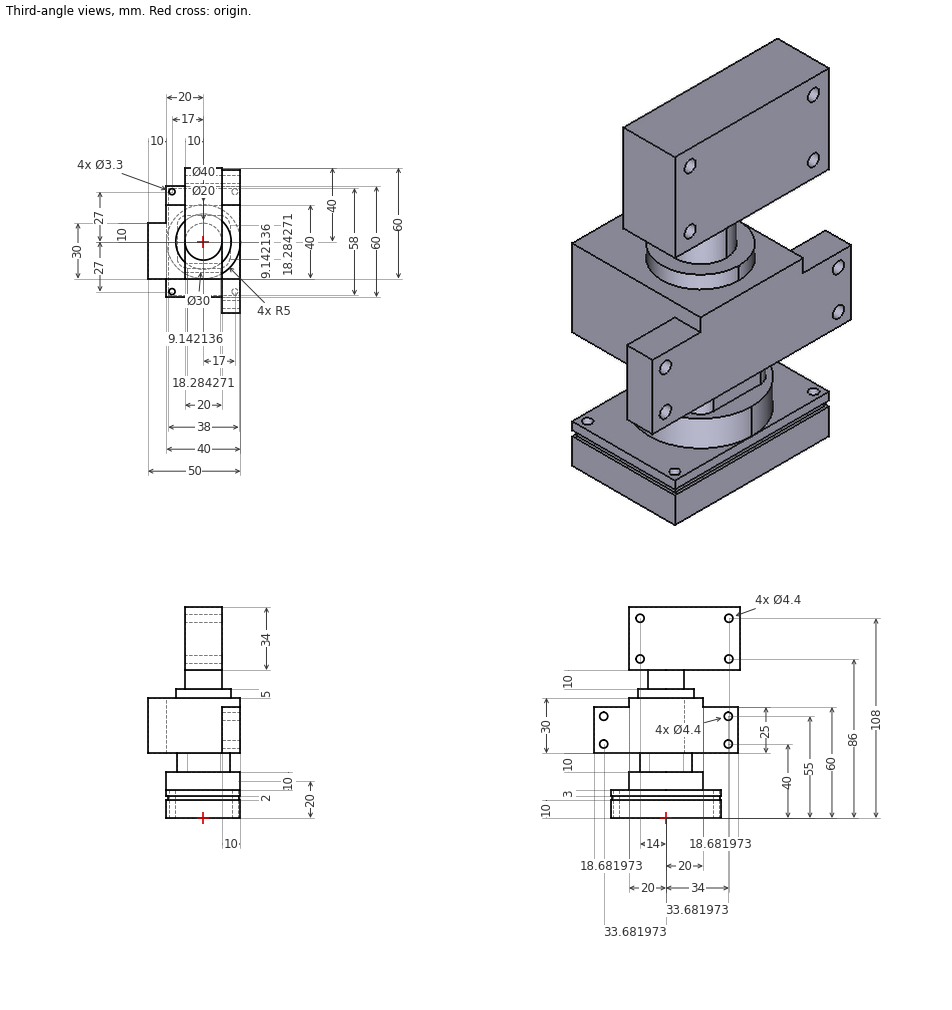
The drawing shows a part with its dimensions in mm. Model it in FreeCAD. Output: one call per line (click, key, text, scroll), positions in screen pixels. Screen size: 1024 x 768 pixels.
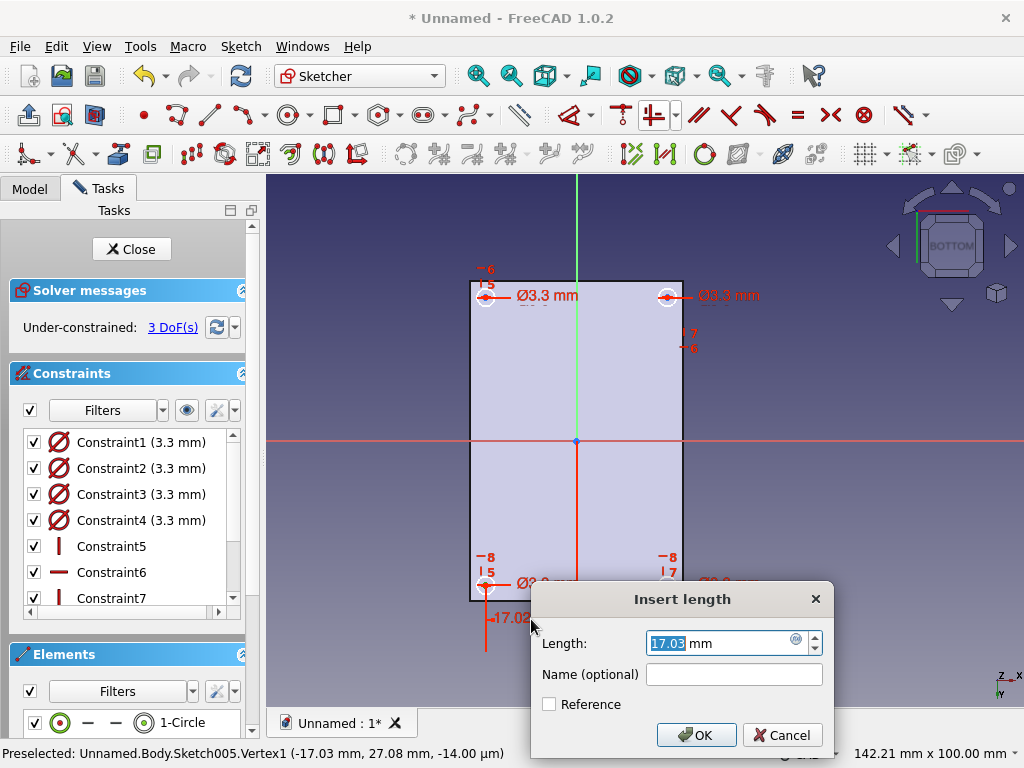
text(17)
key(Return)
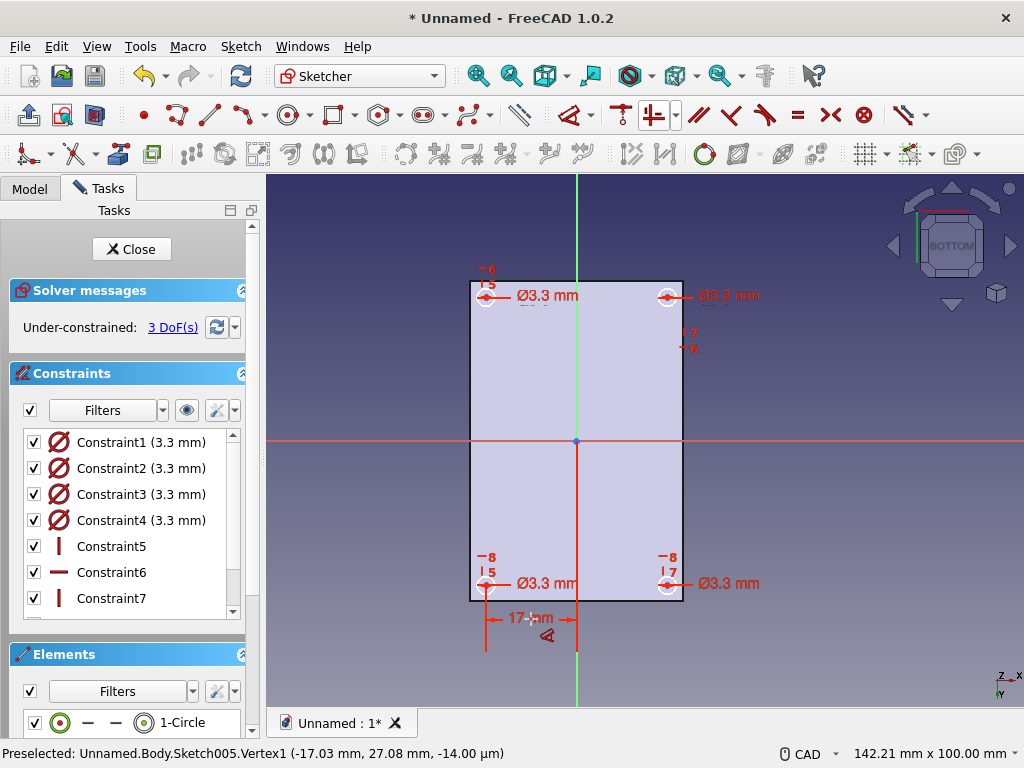
click(486, 585)
click(452, 513)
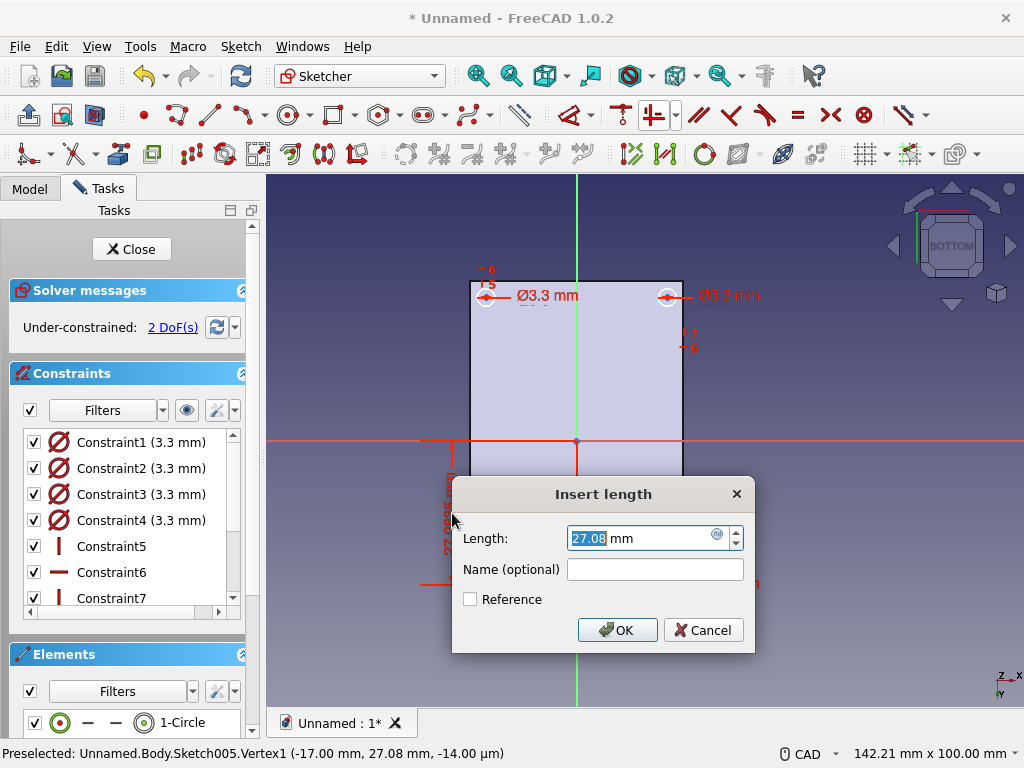
text(27)
key(Return)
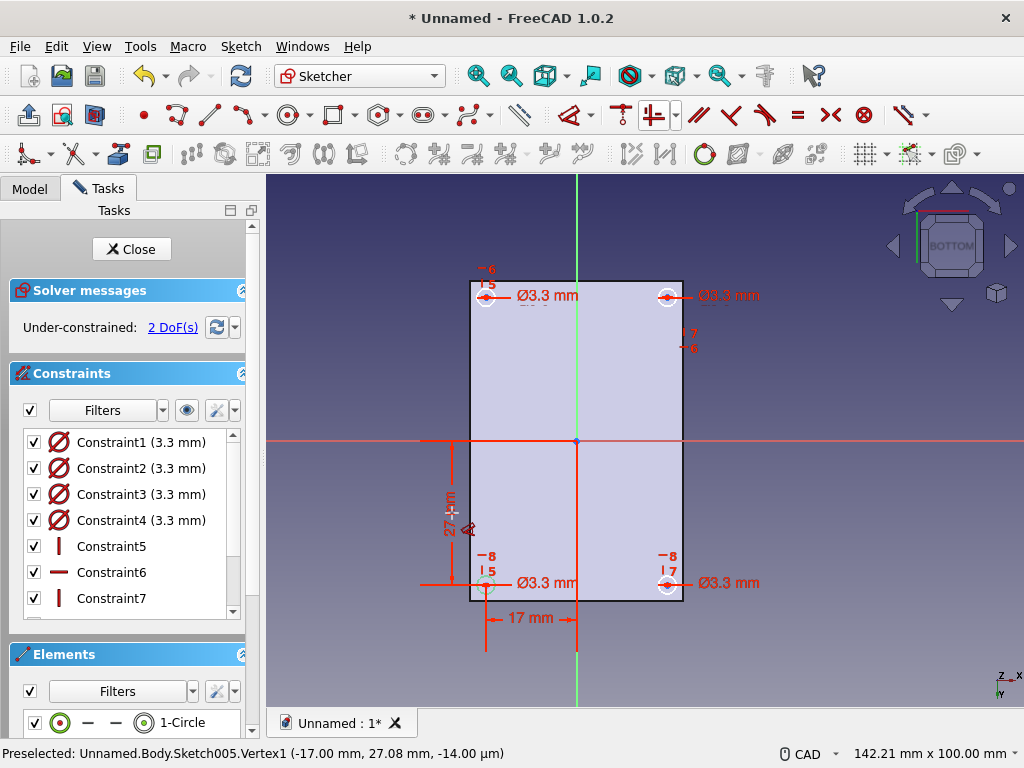
click(486, 298)
click(452, 369)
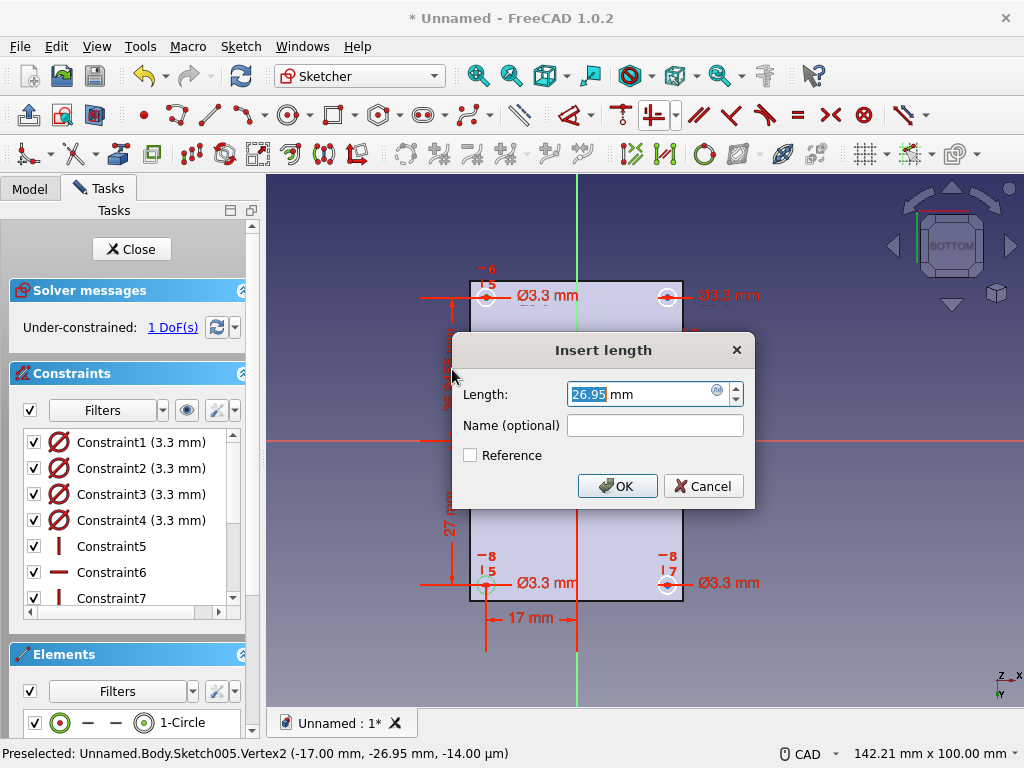
text(27)
key(Return)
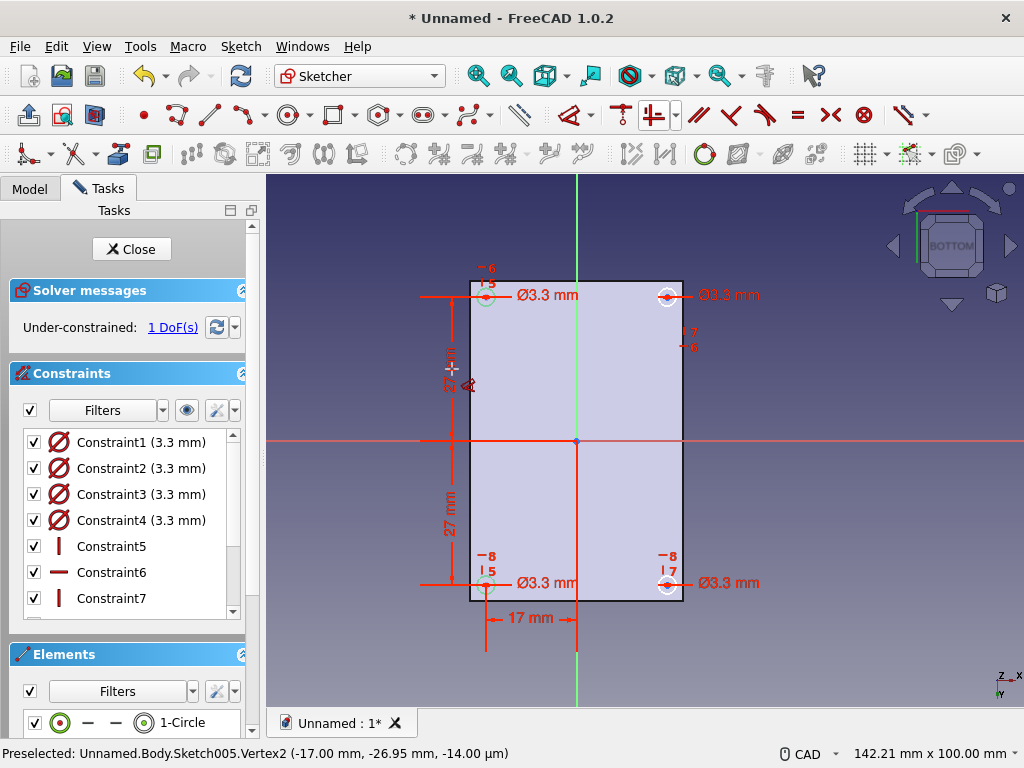
click(667, 297)
click(622, 263)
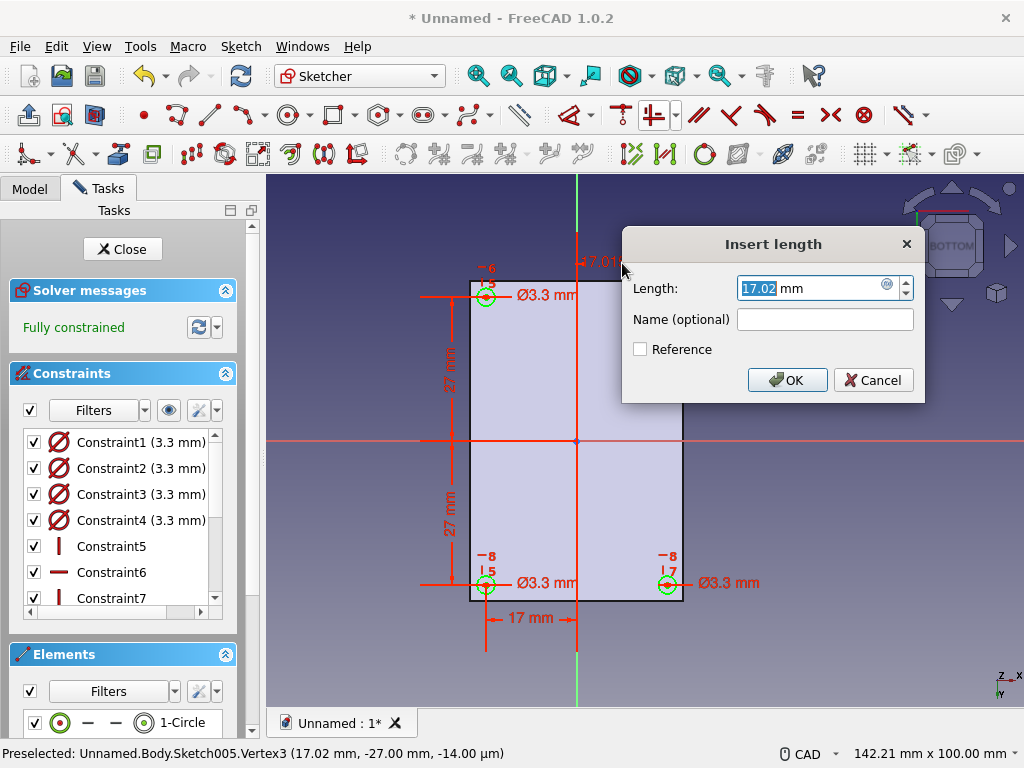
text(17)
key(Return)
key(Escape)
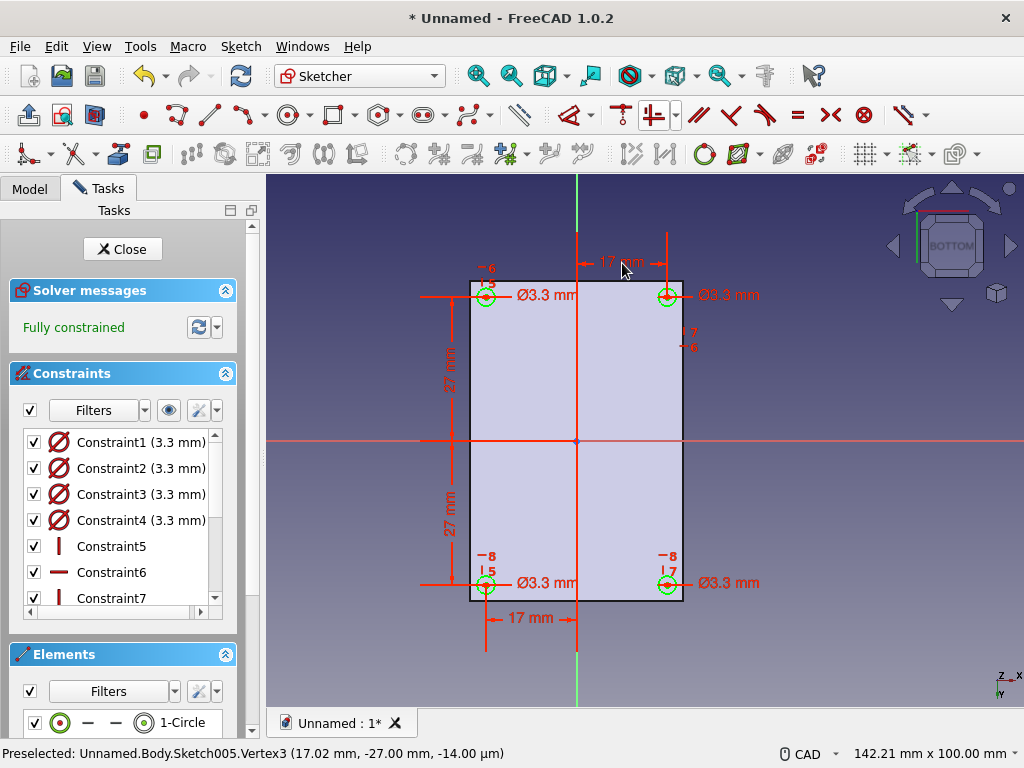
click(123, 249)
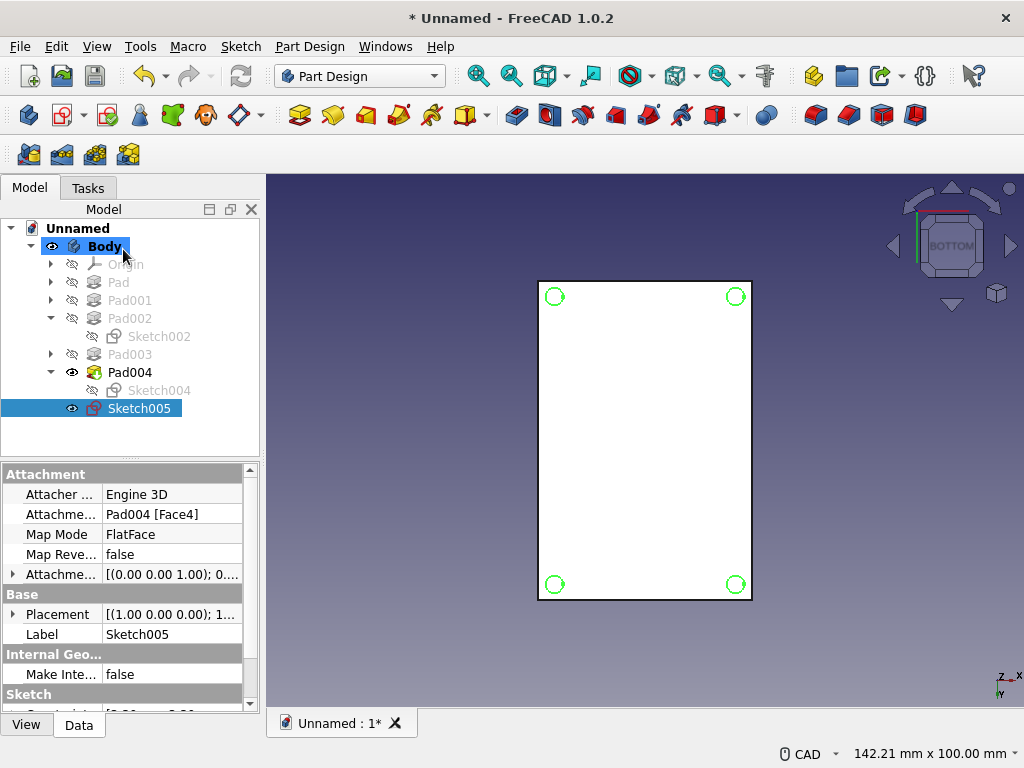
click(517, 116)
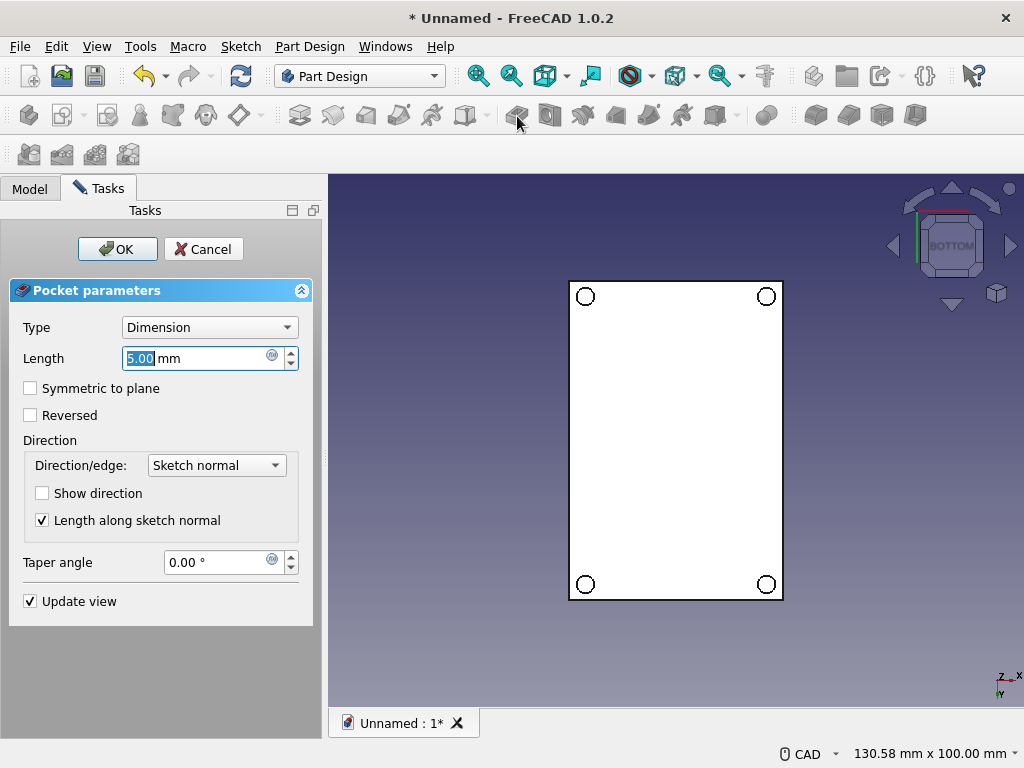
text(20)
key(Tab)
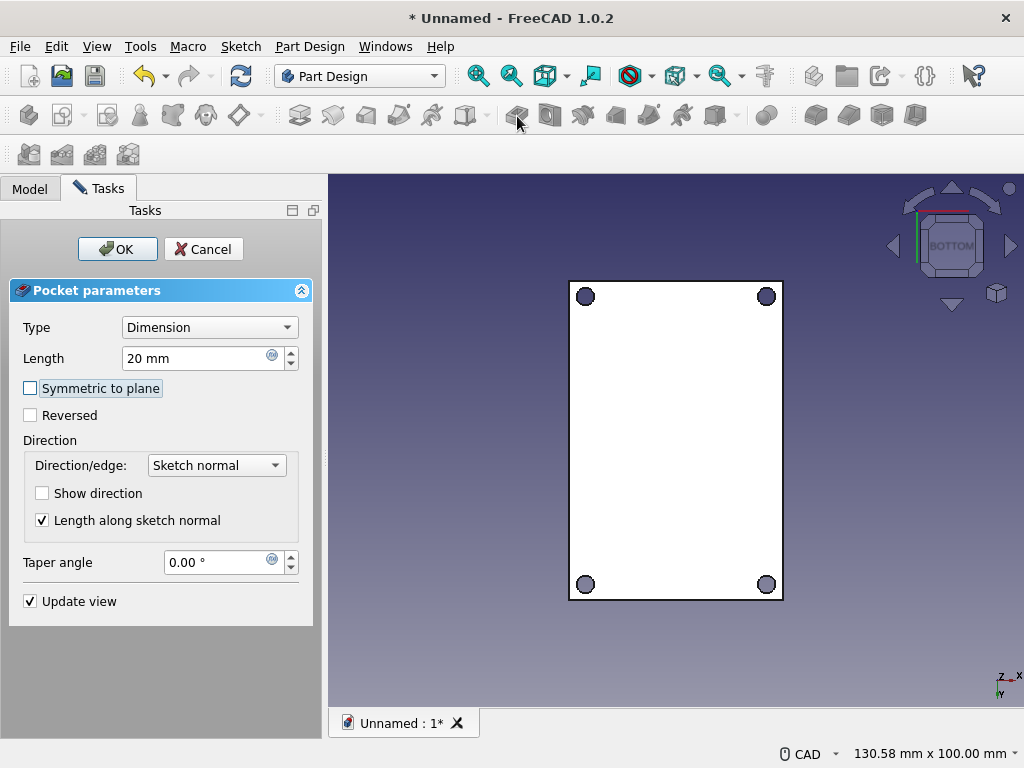
click(118, 249)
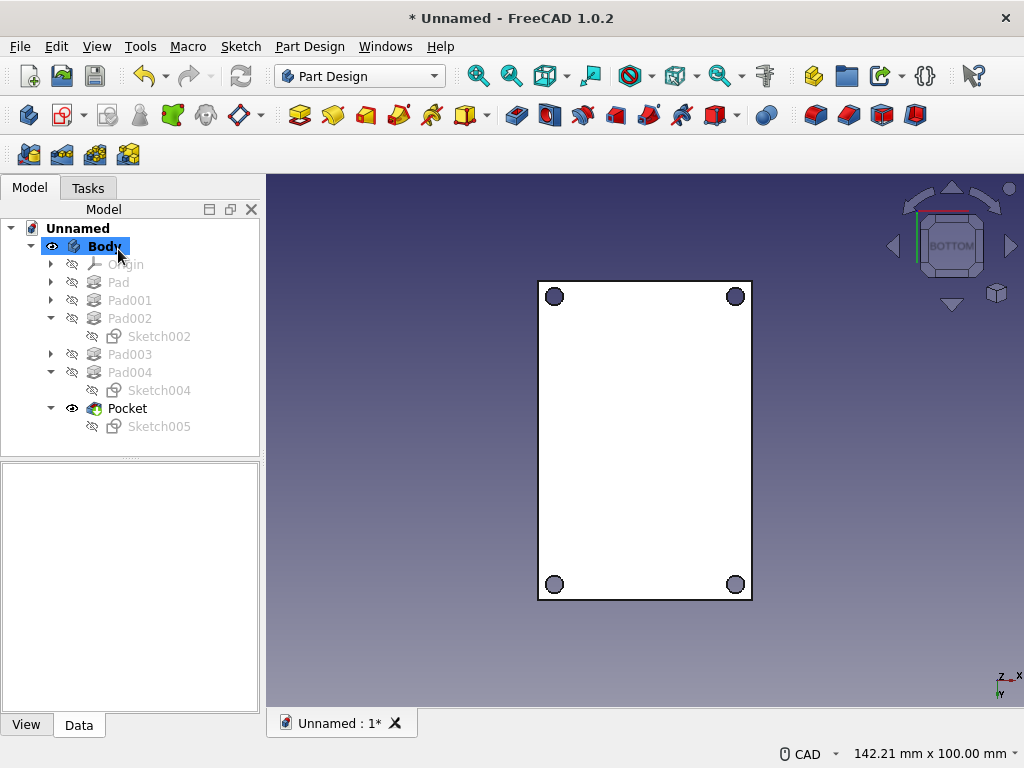
key(0)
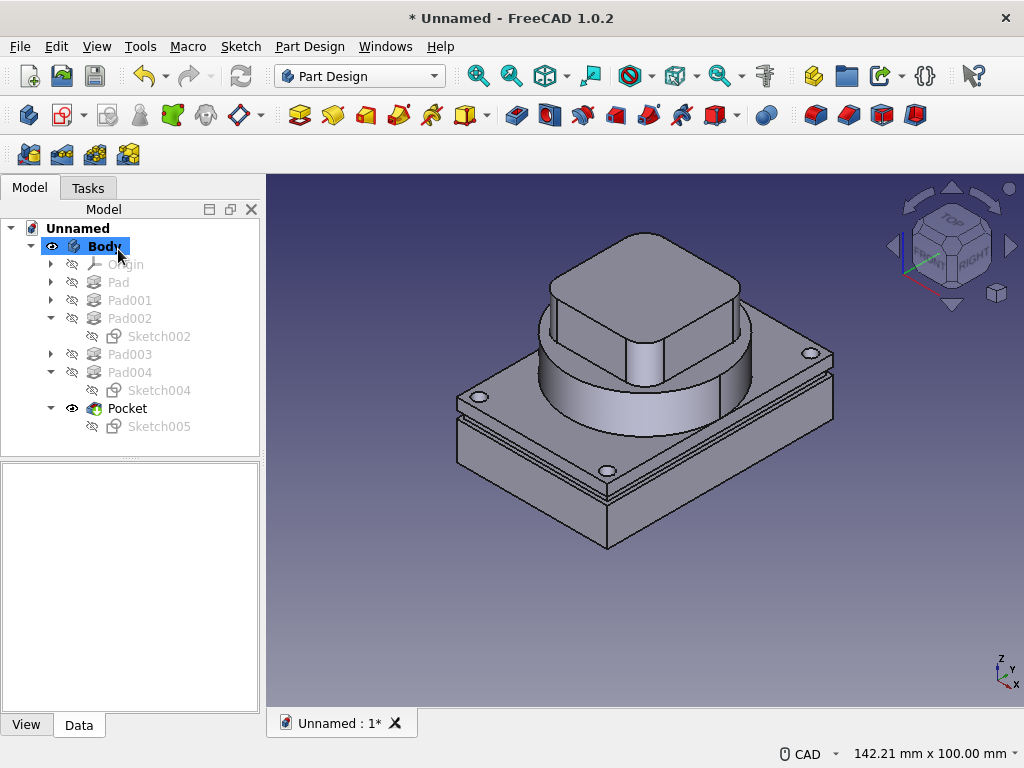
click(645, 287)